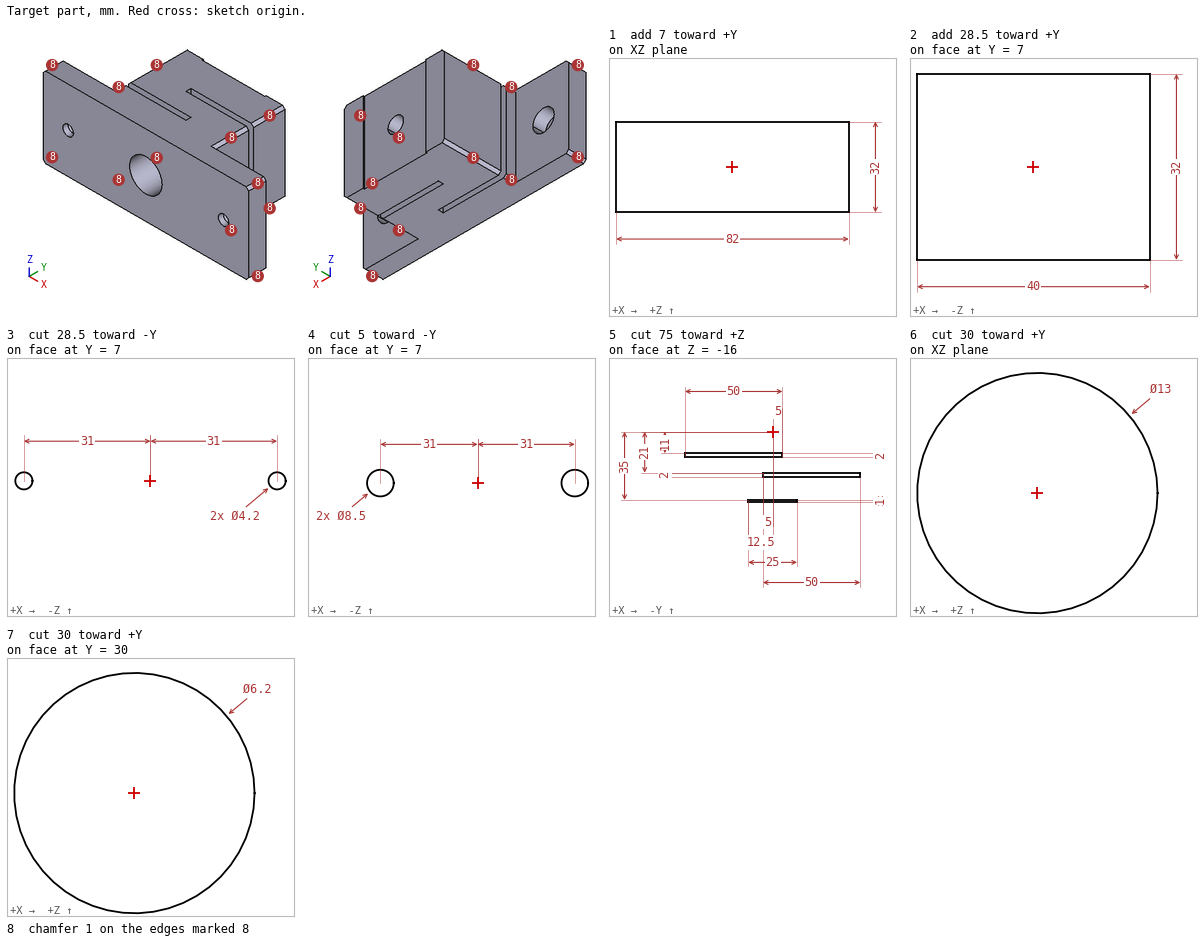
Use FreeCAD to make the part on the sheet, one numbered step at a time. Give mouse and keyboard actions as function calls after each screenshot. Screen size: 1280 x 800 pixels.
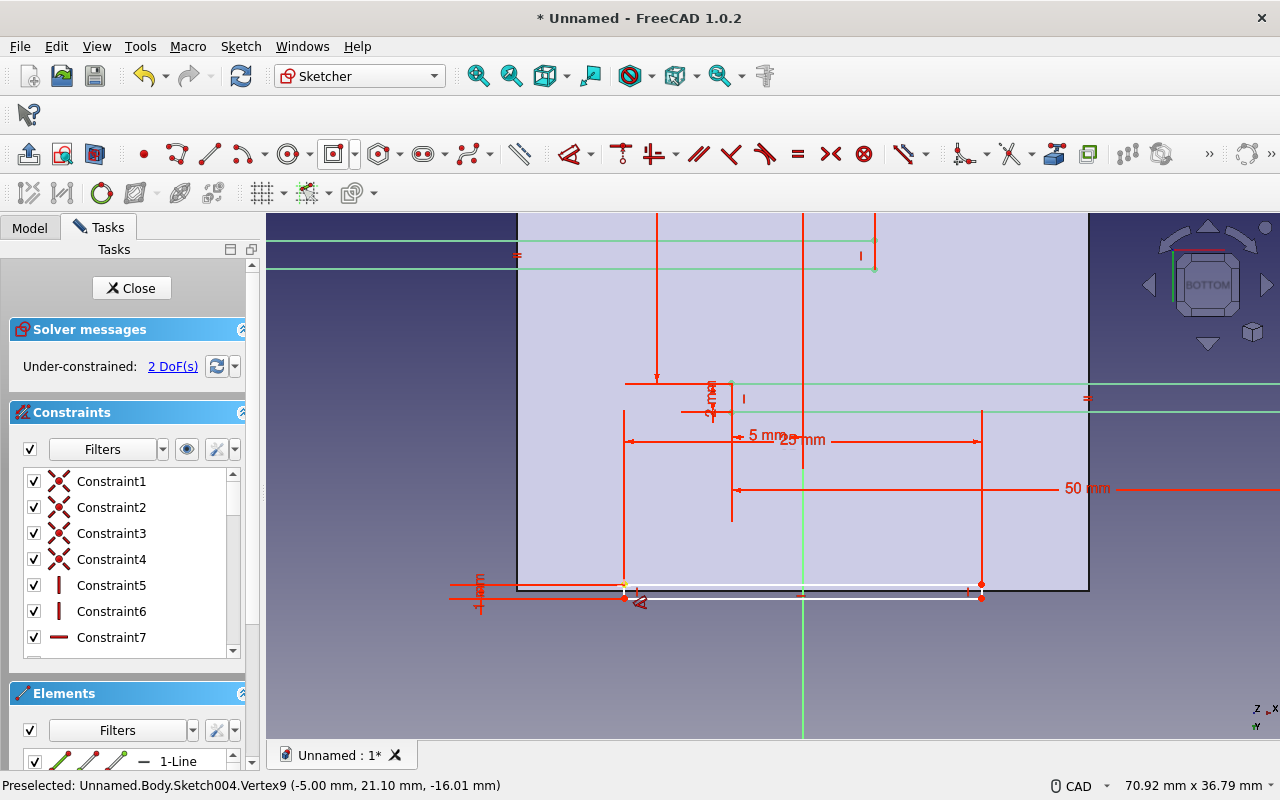
click(624, 585)
click(590, 413)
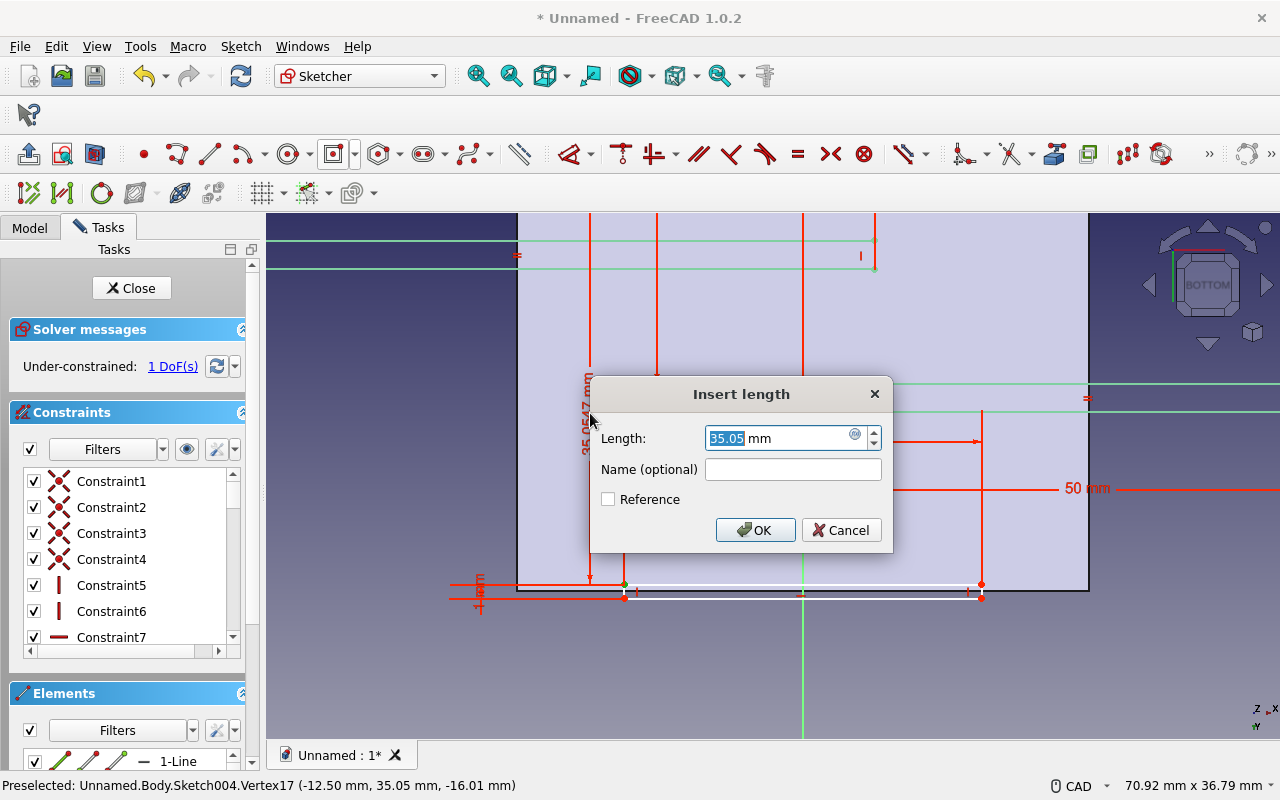
text(35)
key(Return)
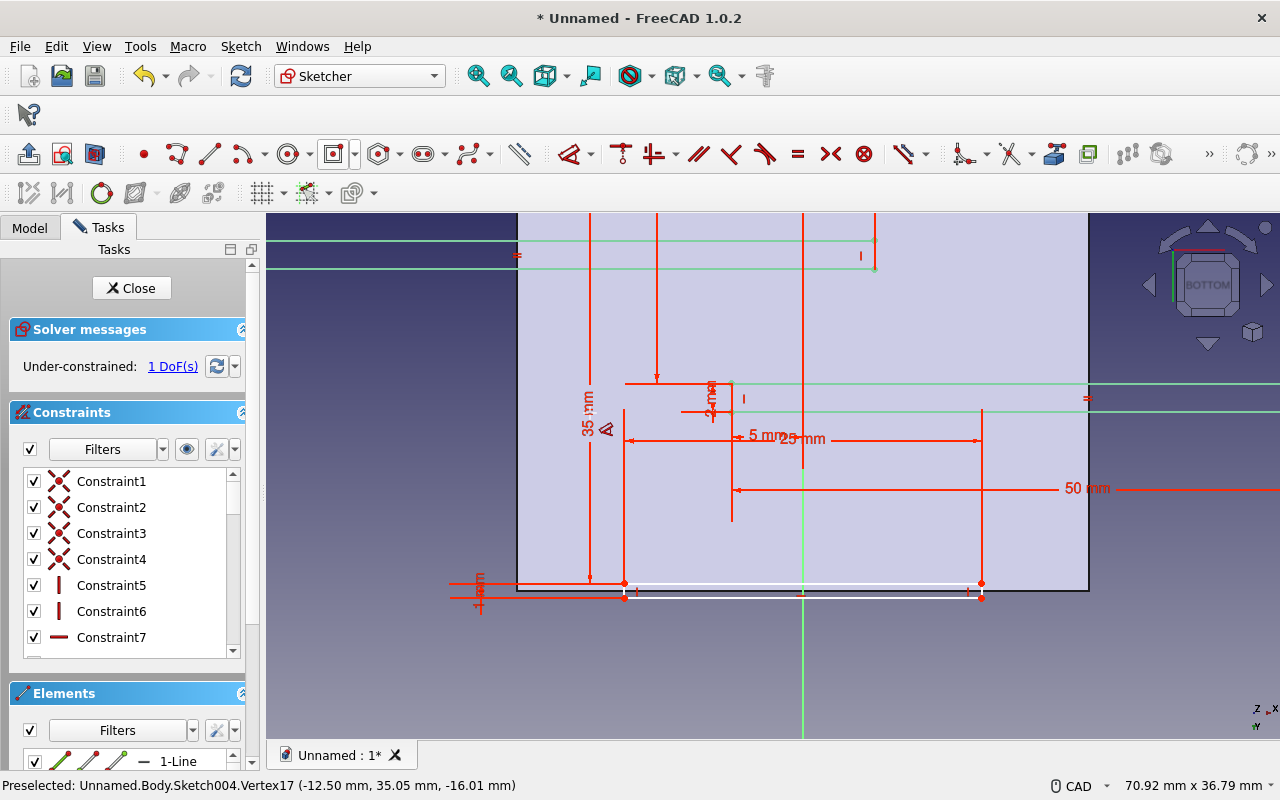
click(624, 584)
click(714, 618)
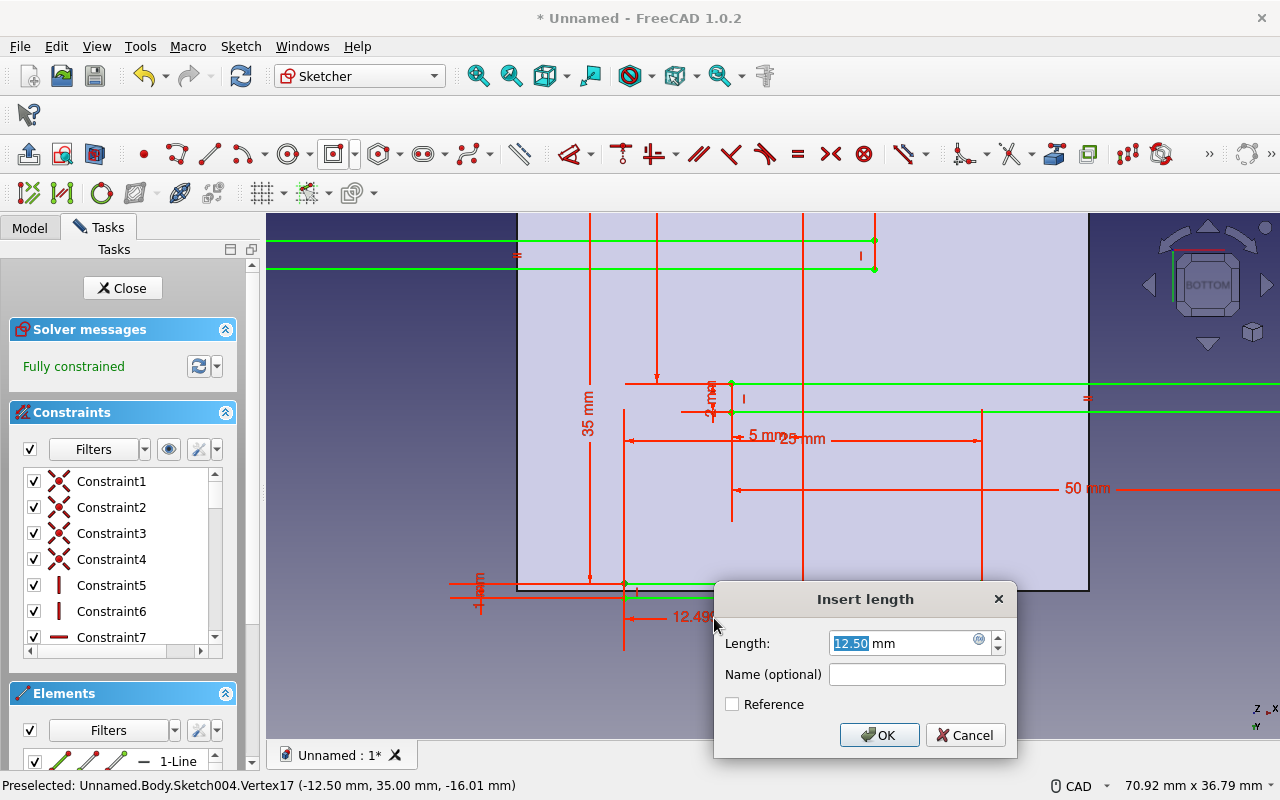
text(12.5)
key(Return)
key(Escape)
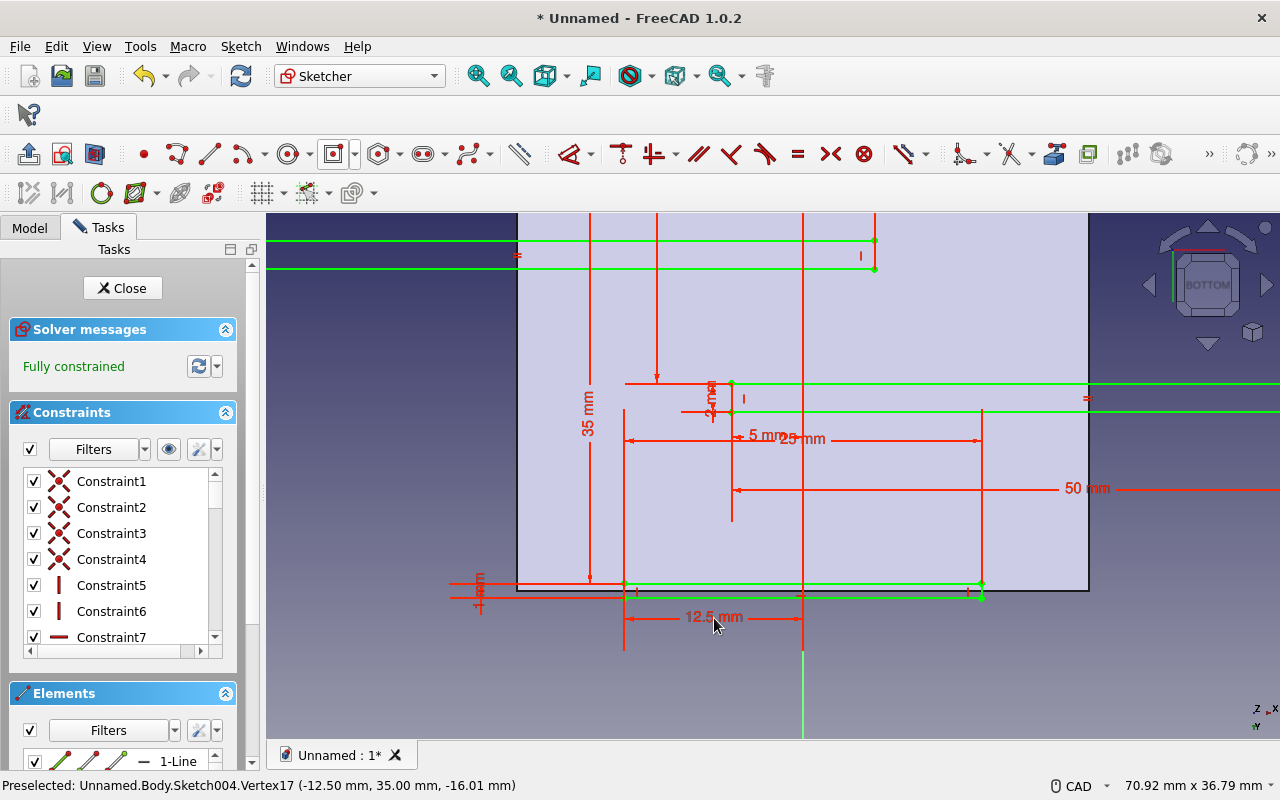
click(123, 288)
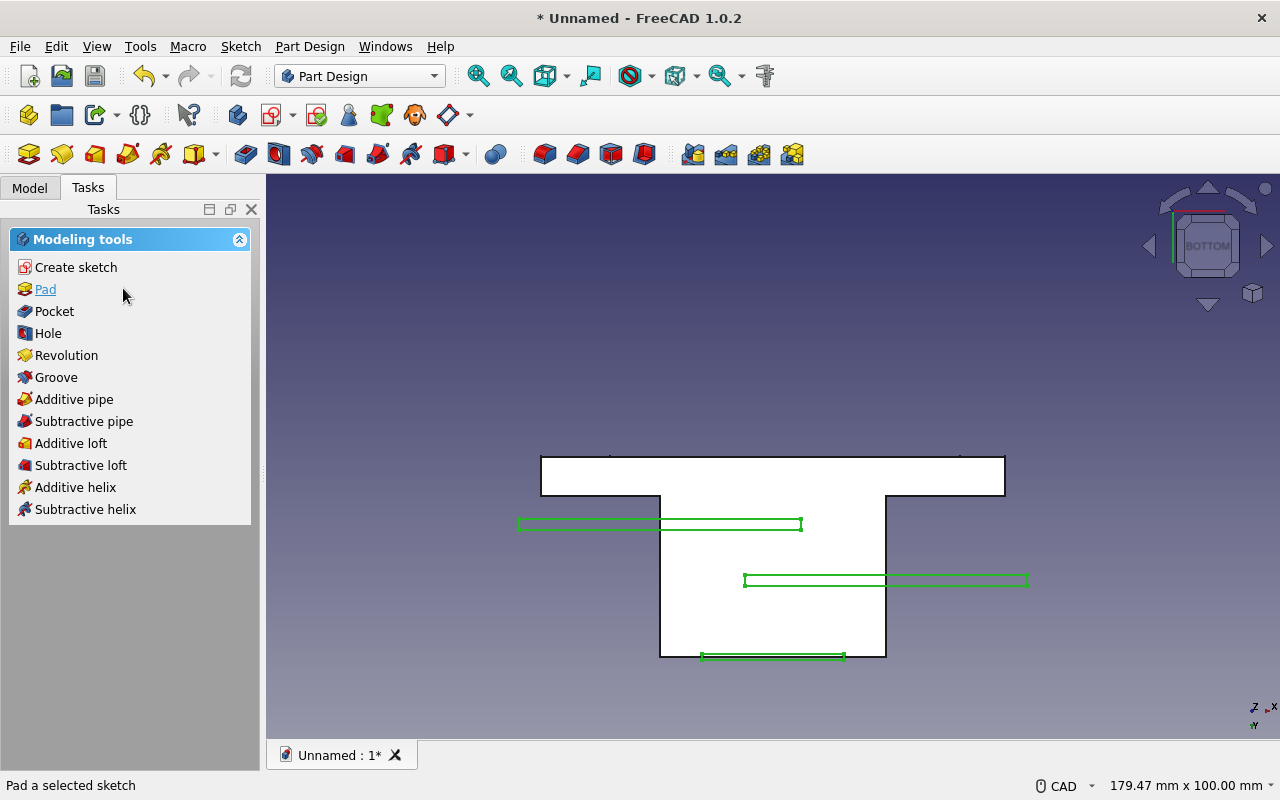
click(246, 154)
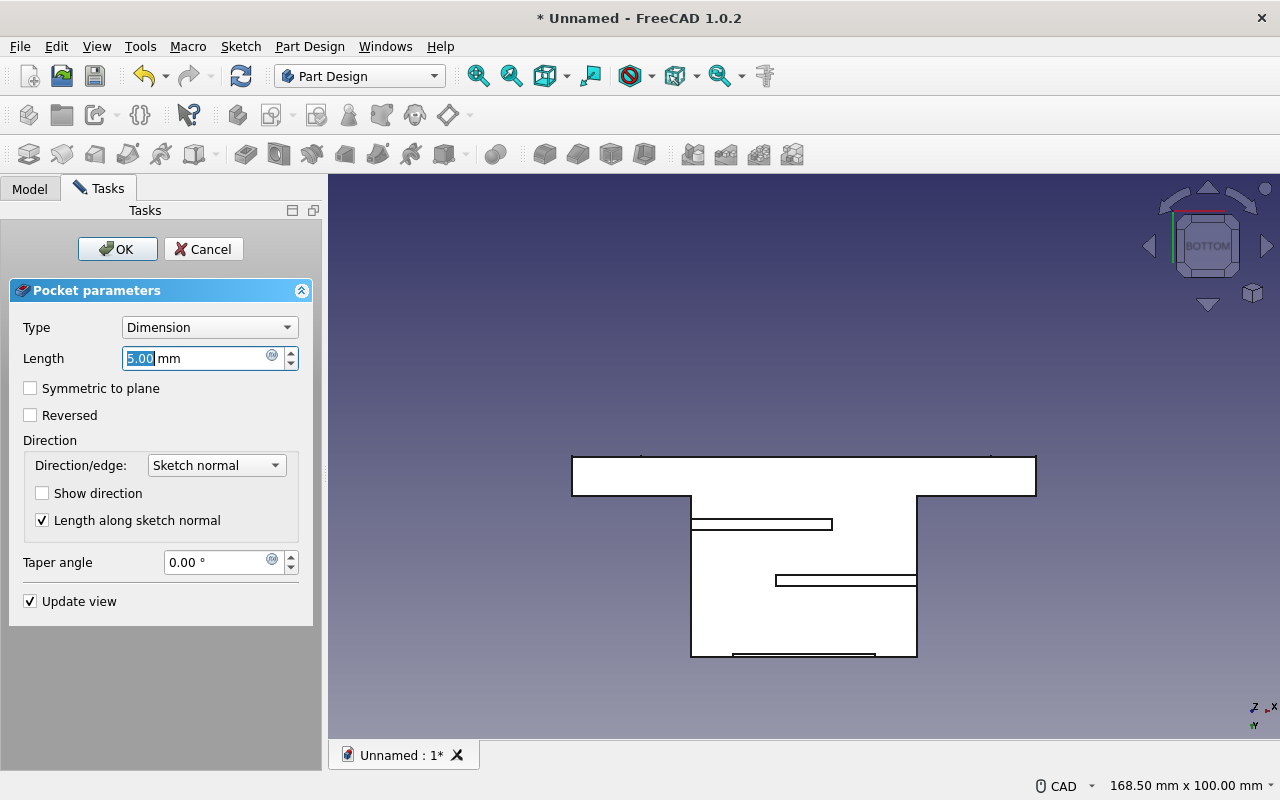
text(75)
key(Tab)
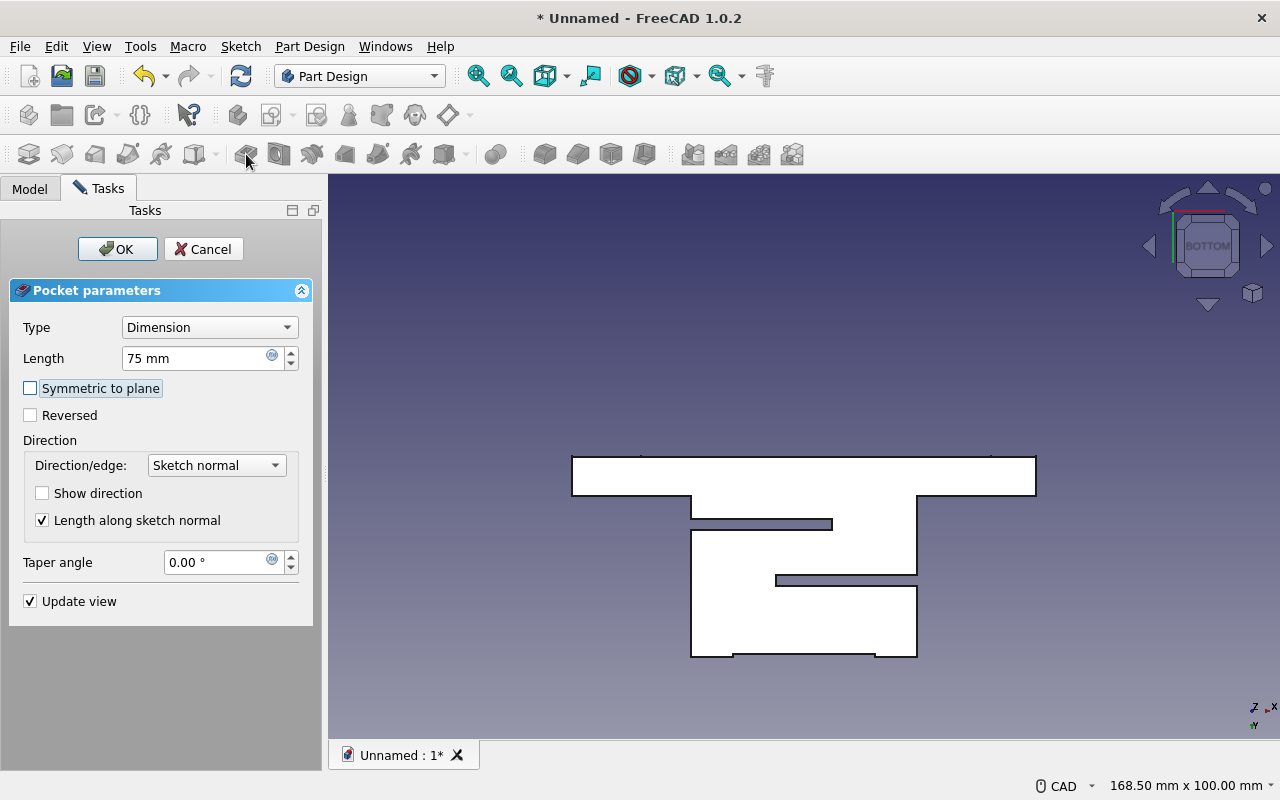
click(118, 249)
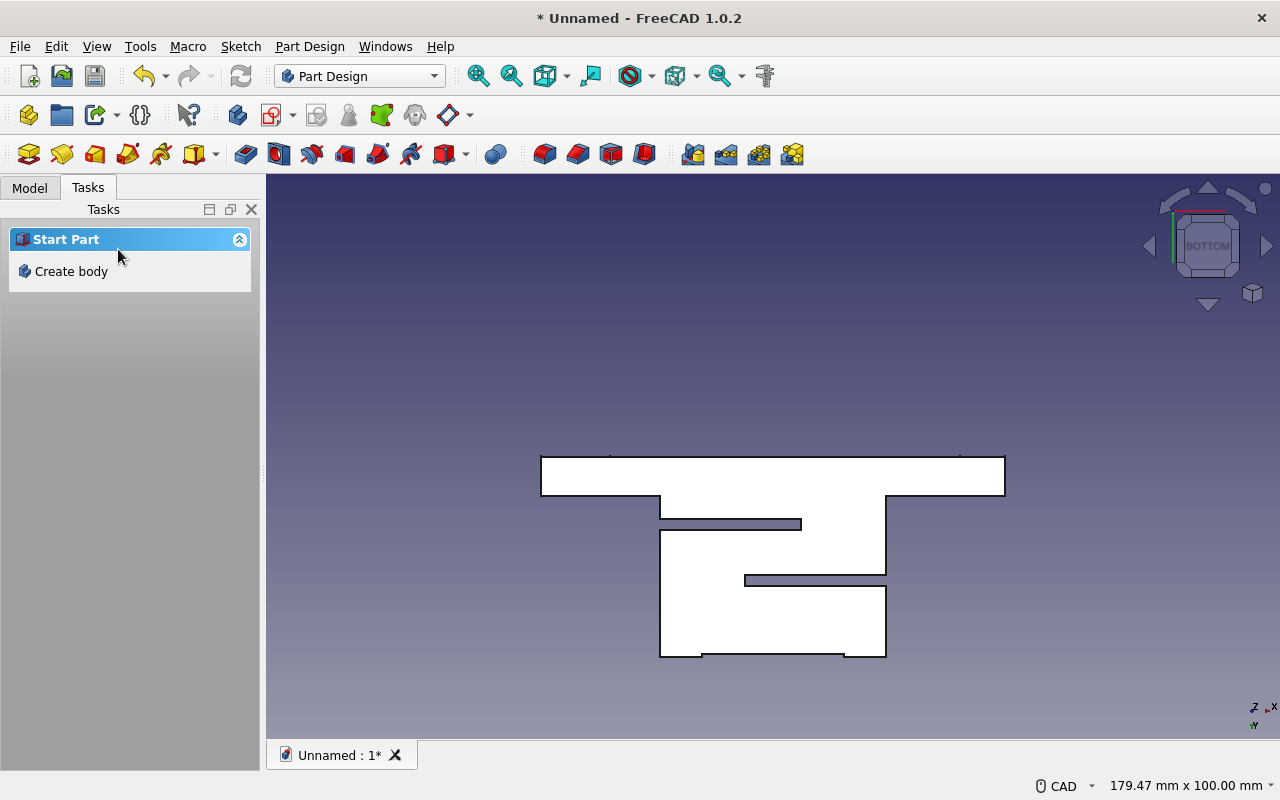
click(270, 116)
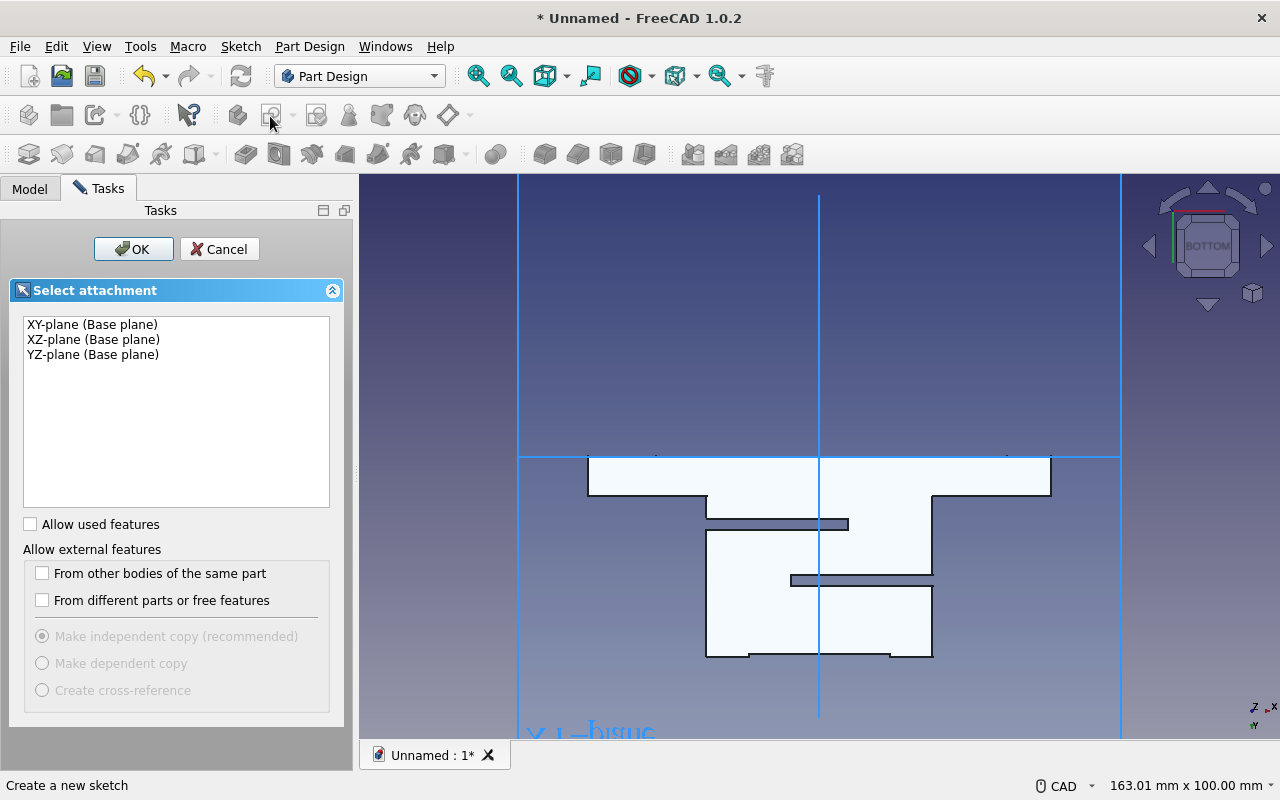
click(84, 340)